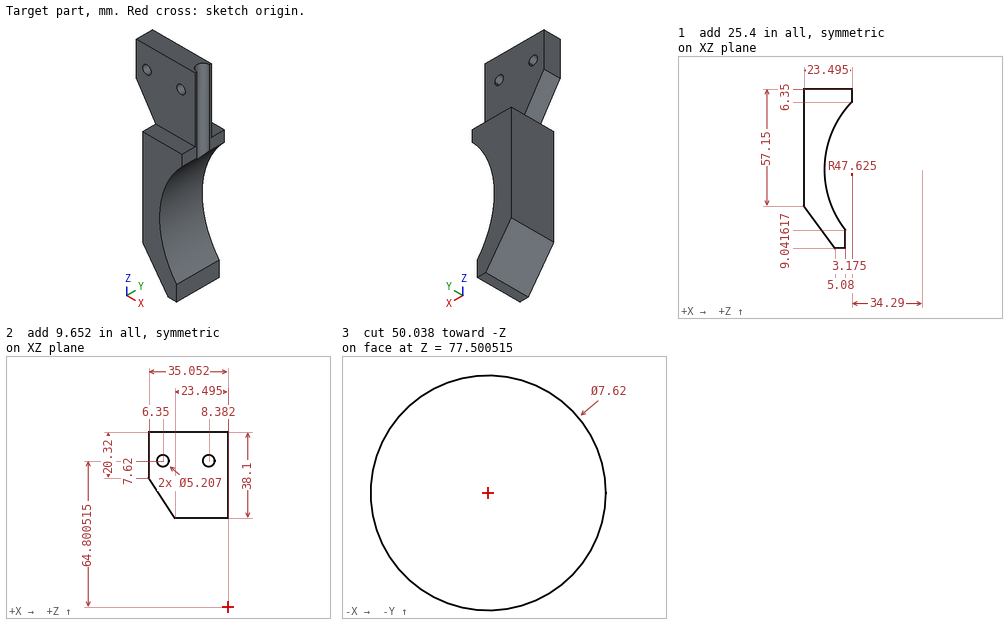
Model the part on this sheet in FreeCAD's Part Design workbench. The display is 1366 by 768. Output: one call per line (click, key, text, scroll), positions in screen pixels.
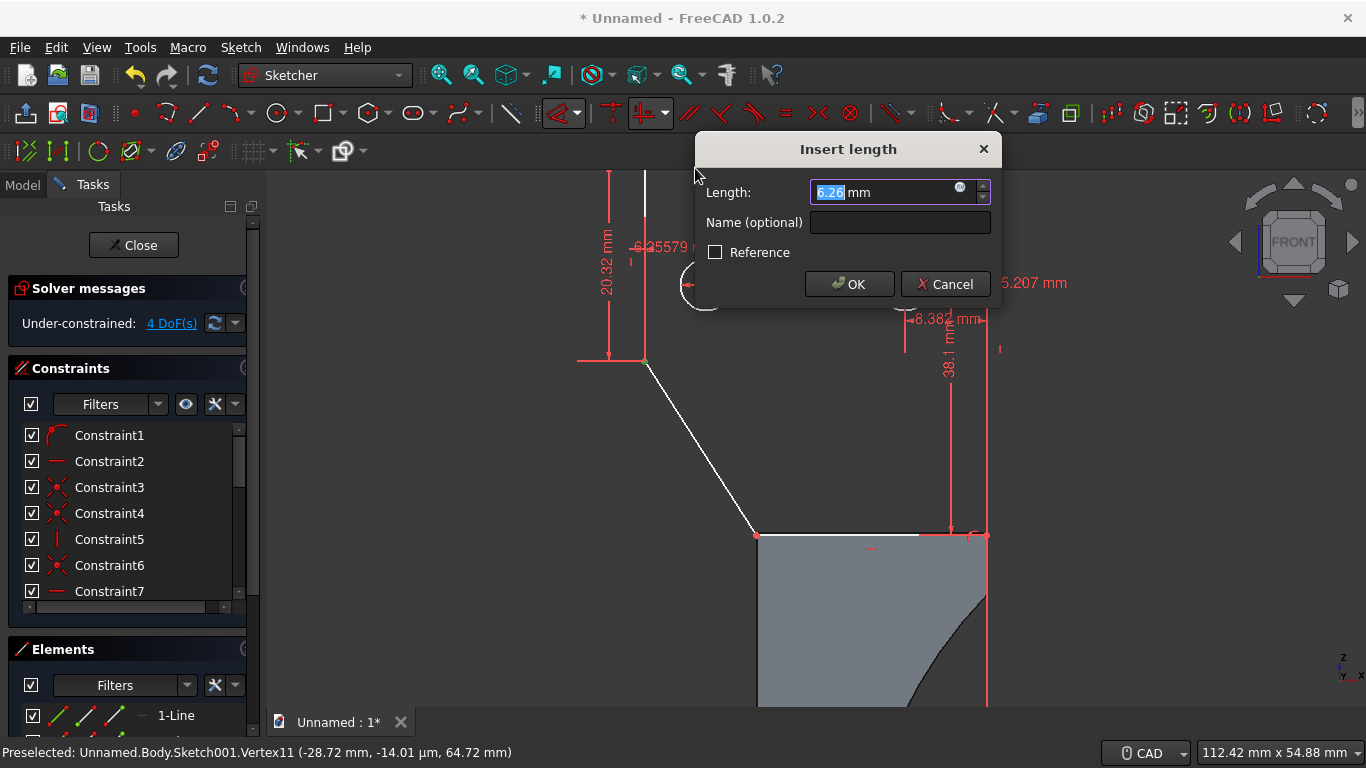
text(6.35)
key(Return)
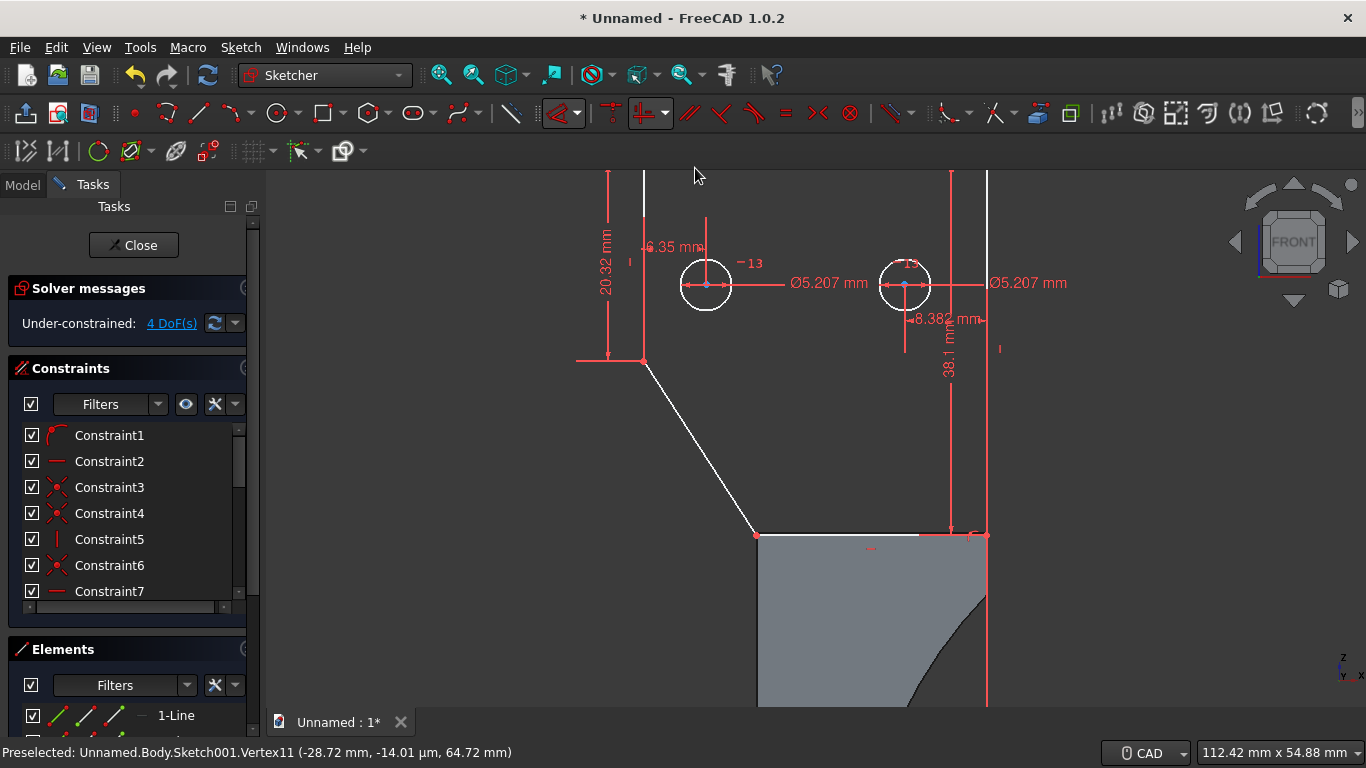
click(644, 361)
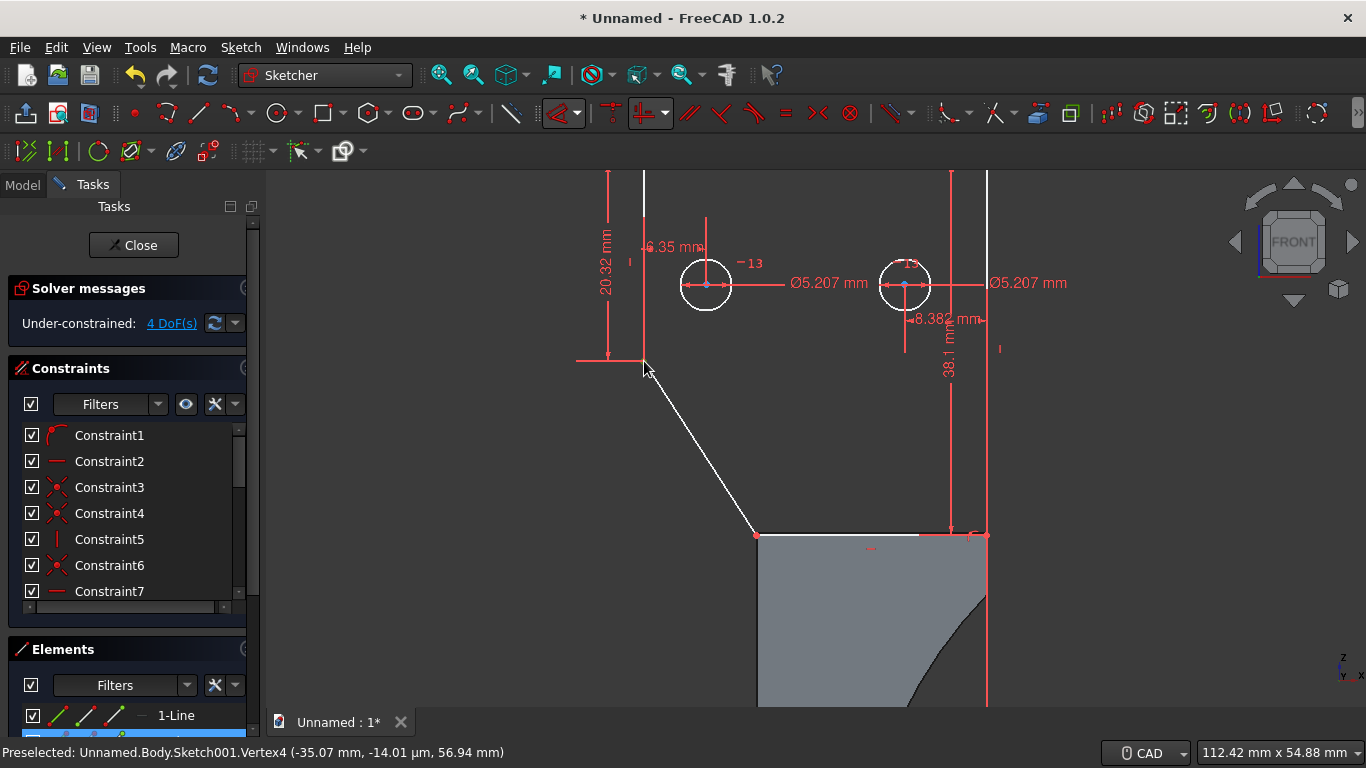
click(706, 285)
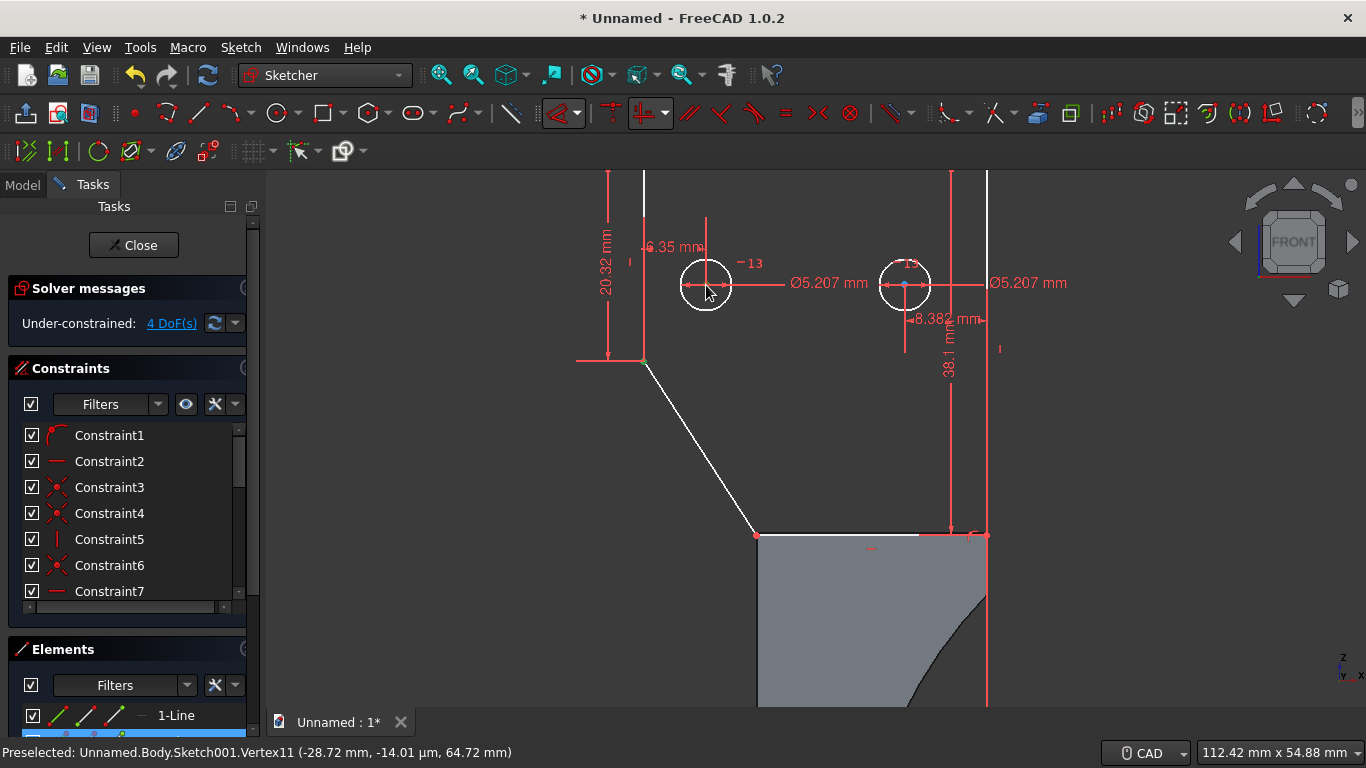
click(580, 114)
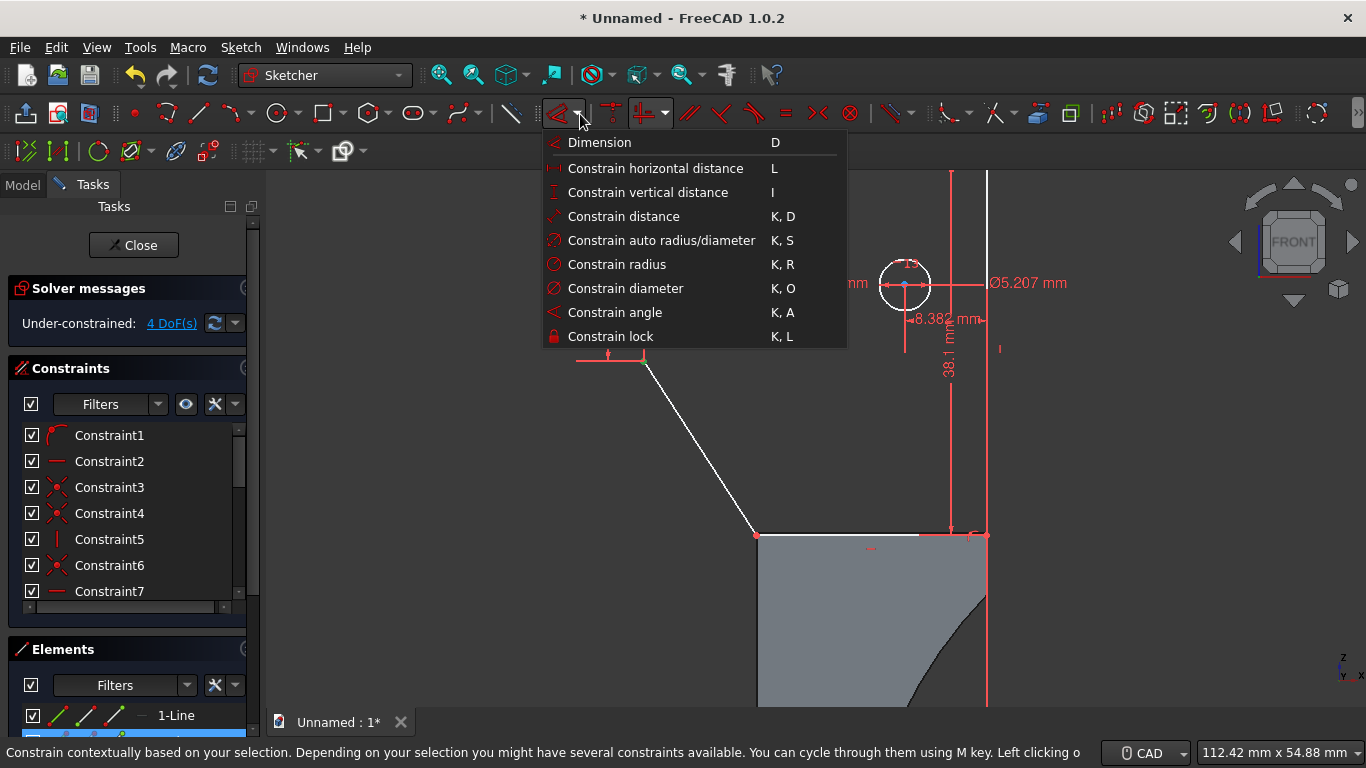
click(695, 192)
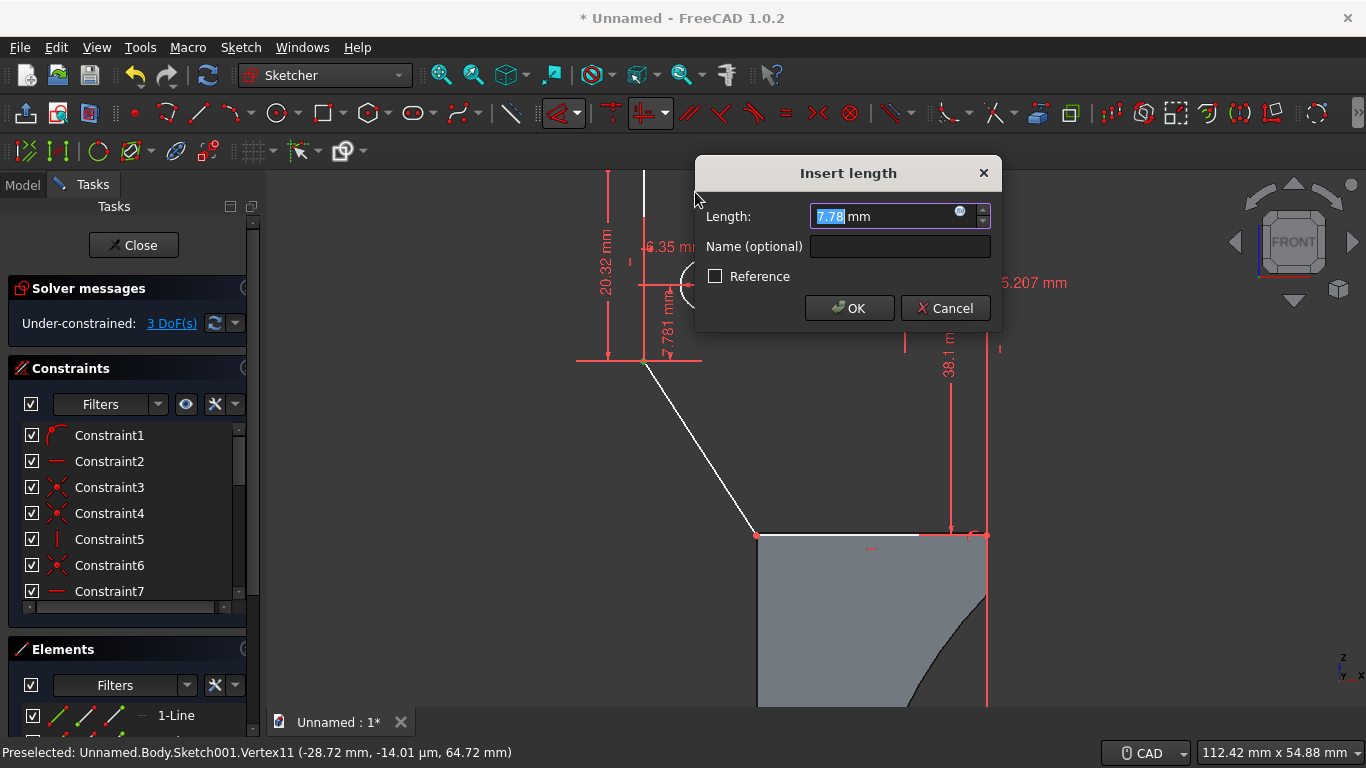
text(7.62)
key(Return)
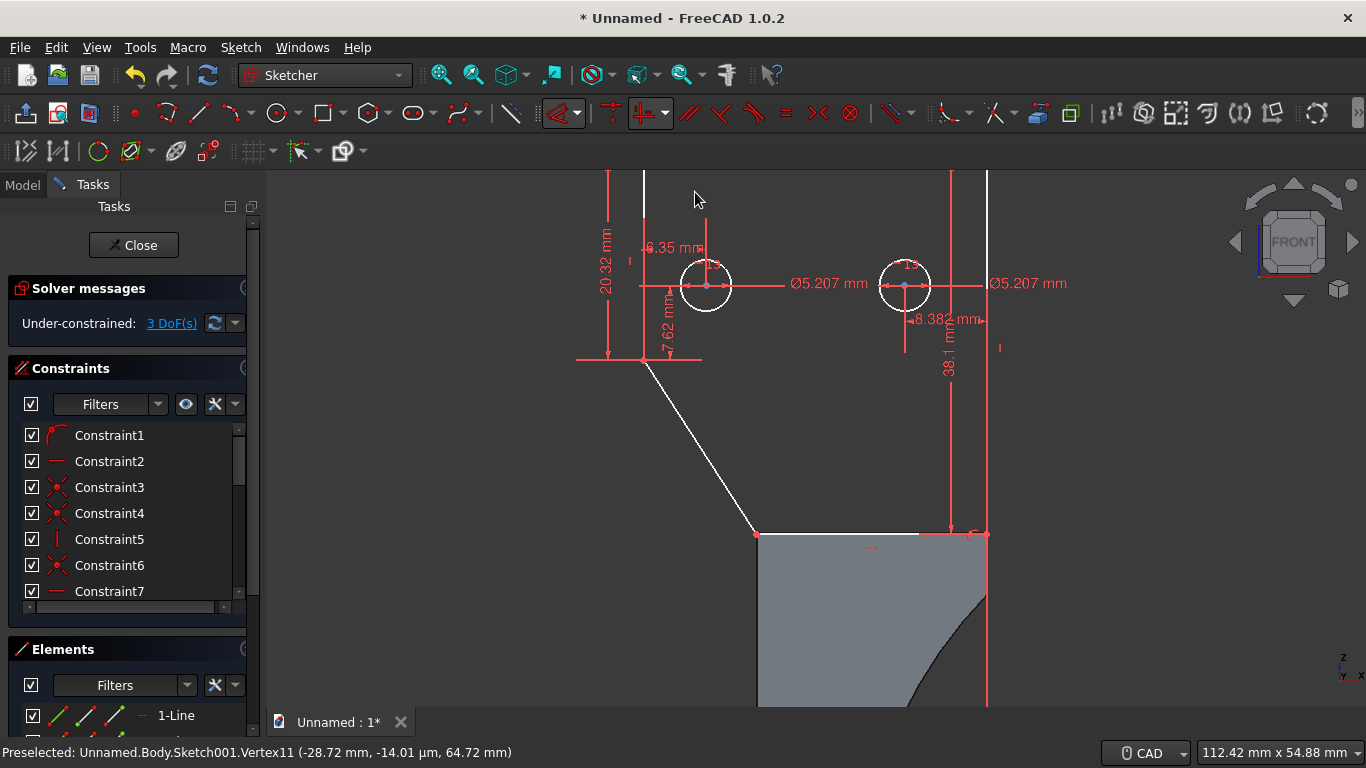
click(918, 534)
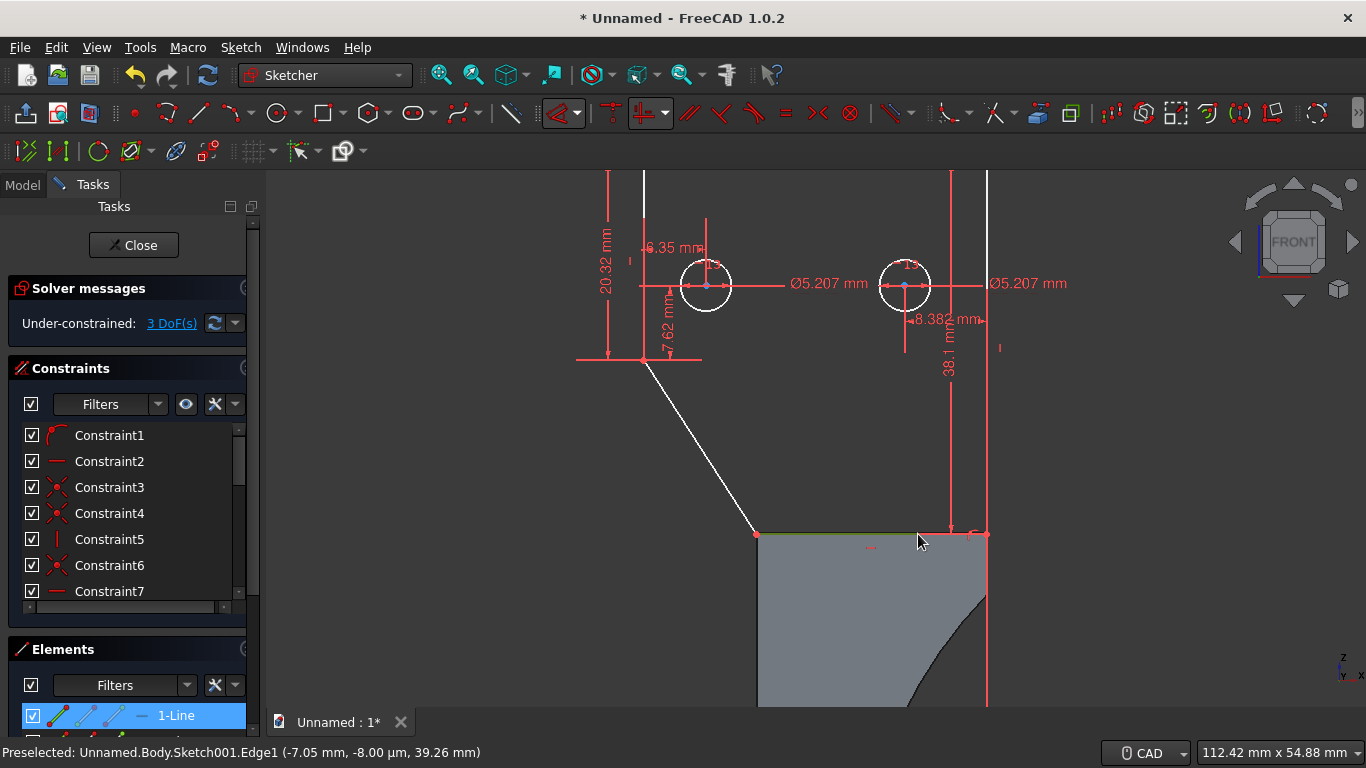
click(580, 114)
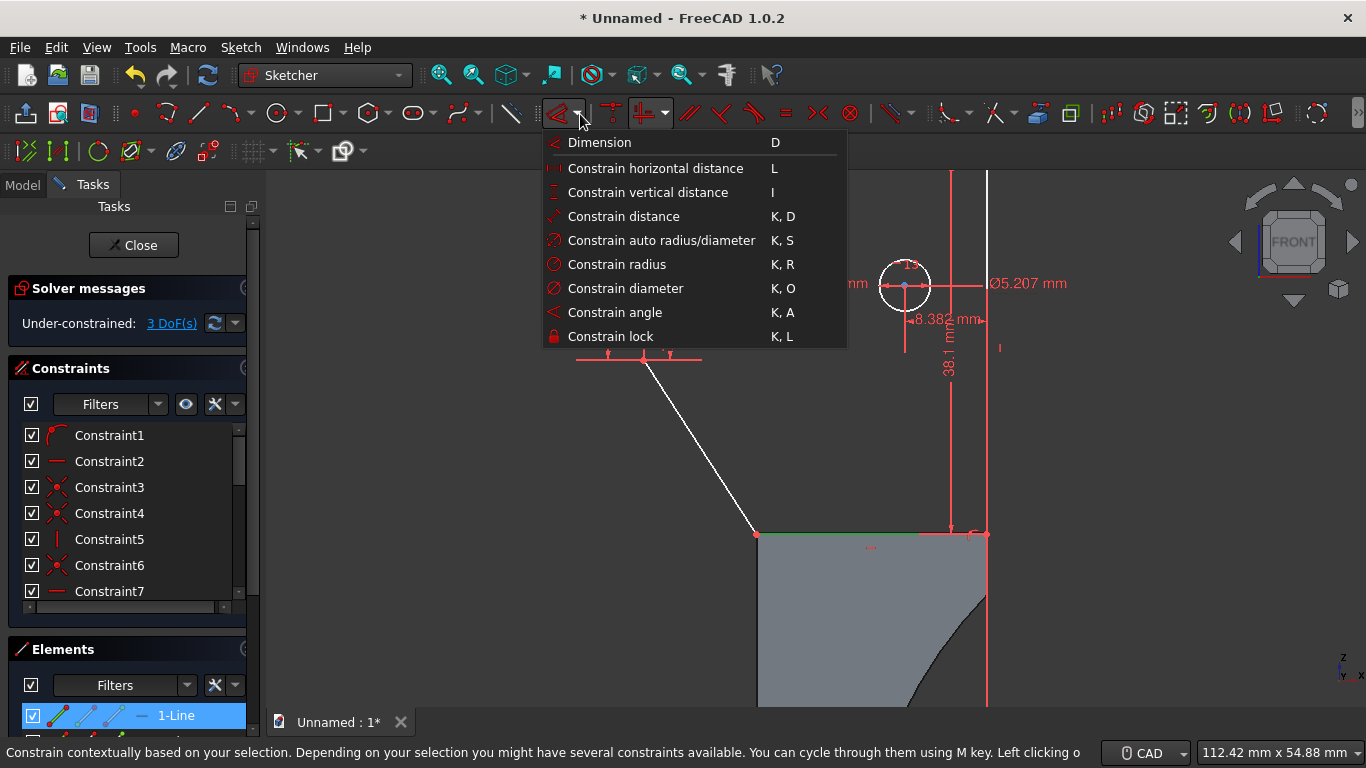
click(695, 168)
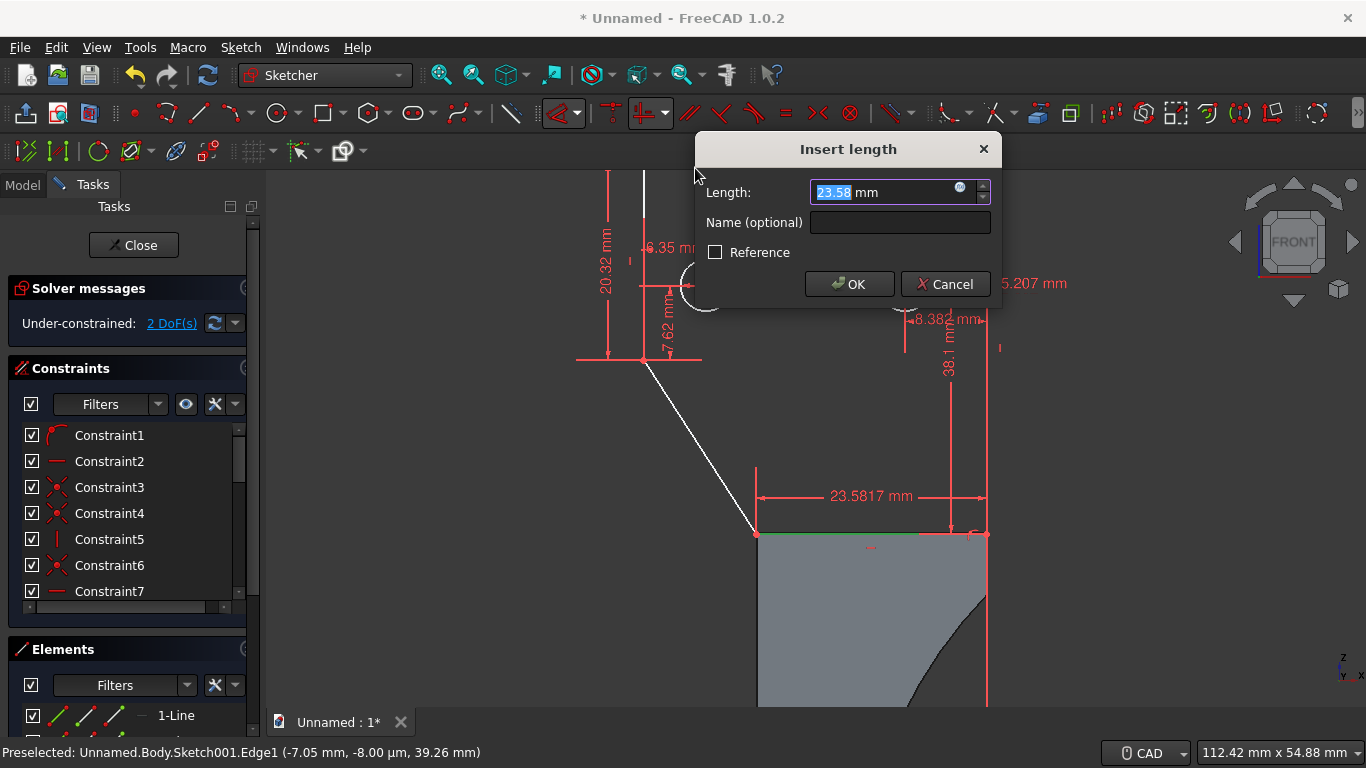
text(23.495)
key(Return)